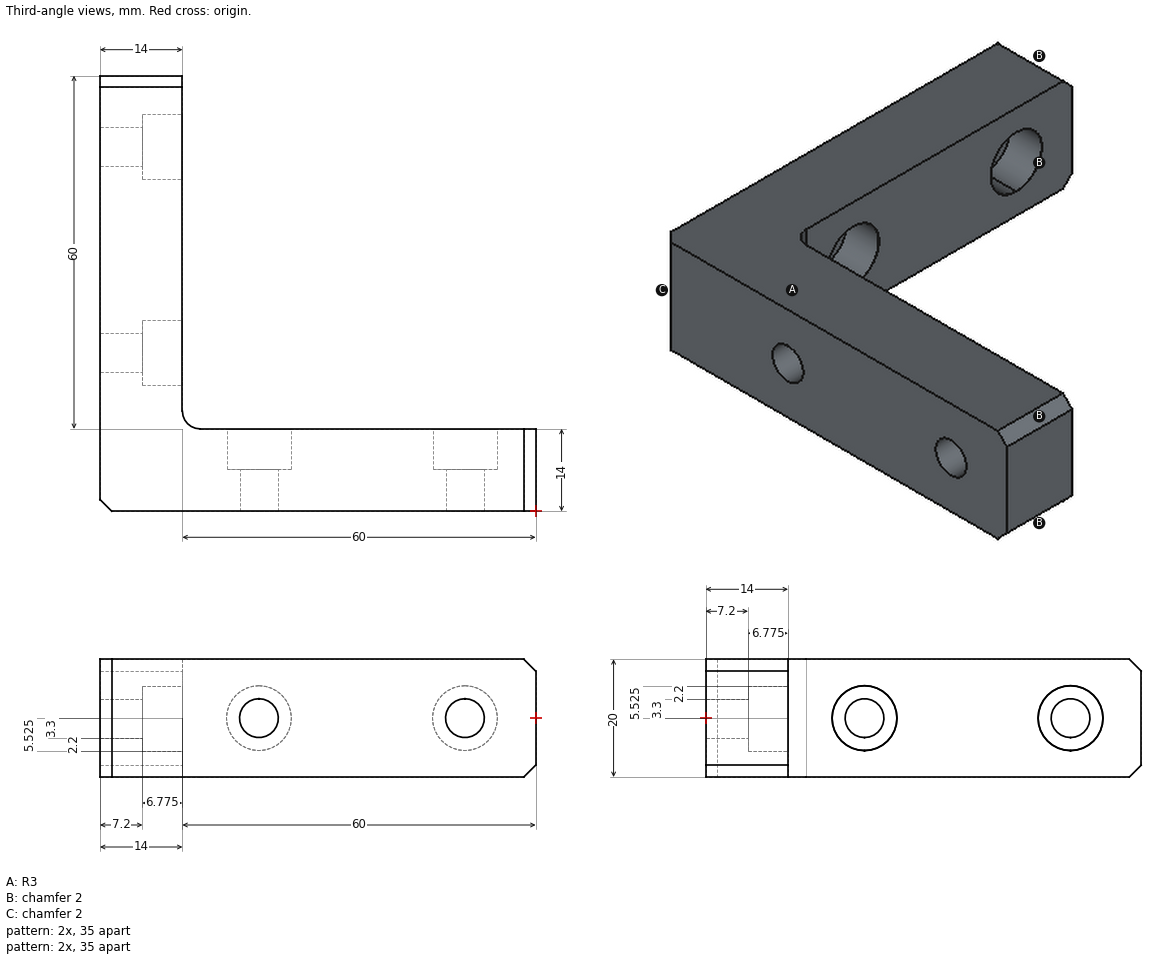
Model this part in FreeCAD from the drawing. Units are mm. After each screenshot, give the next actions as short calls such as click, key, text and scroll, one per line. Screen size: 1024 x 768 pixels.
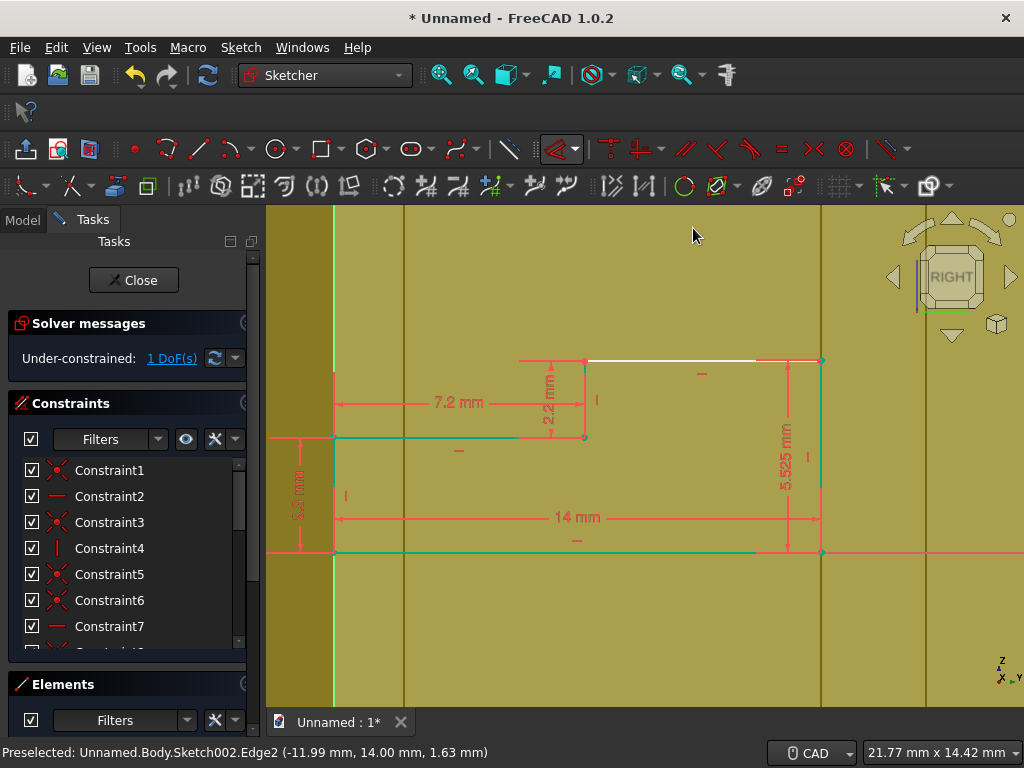
click(750, 361)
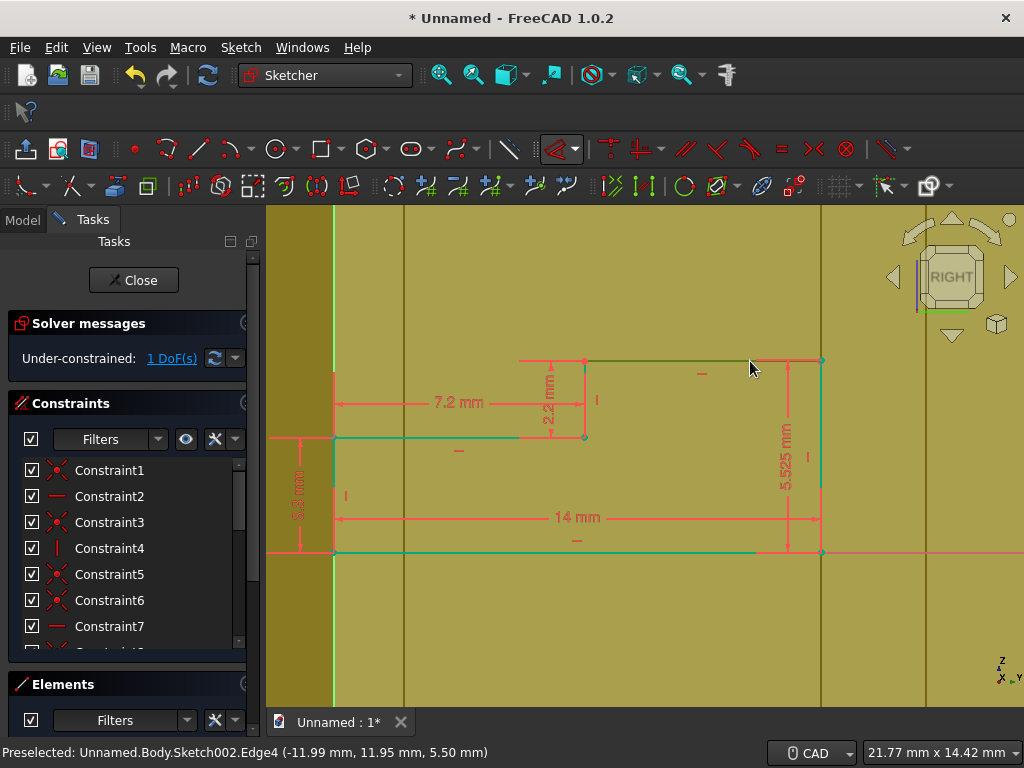
click(578, 150)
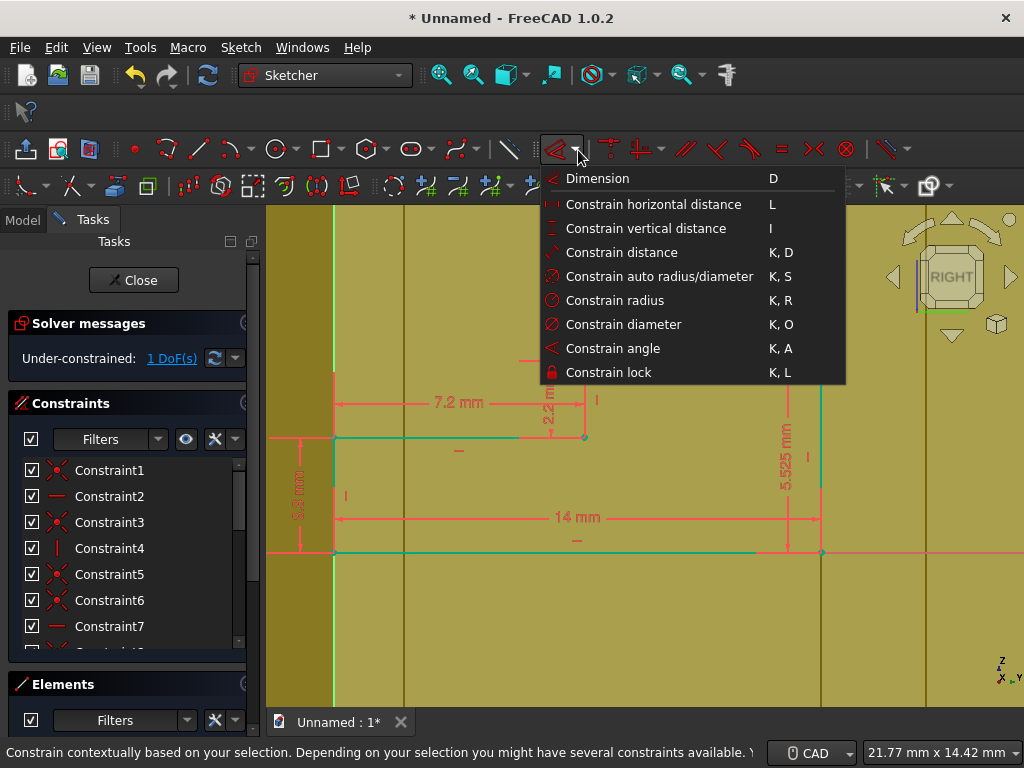
click(693, 204)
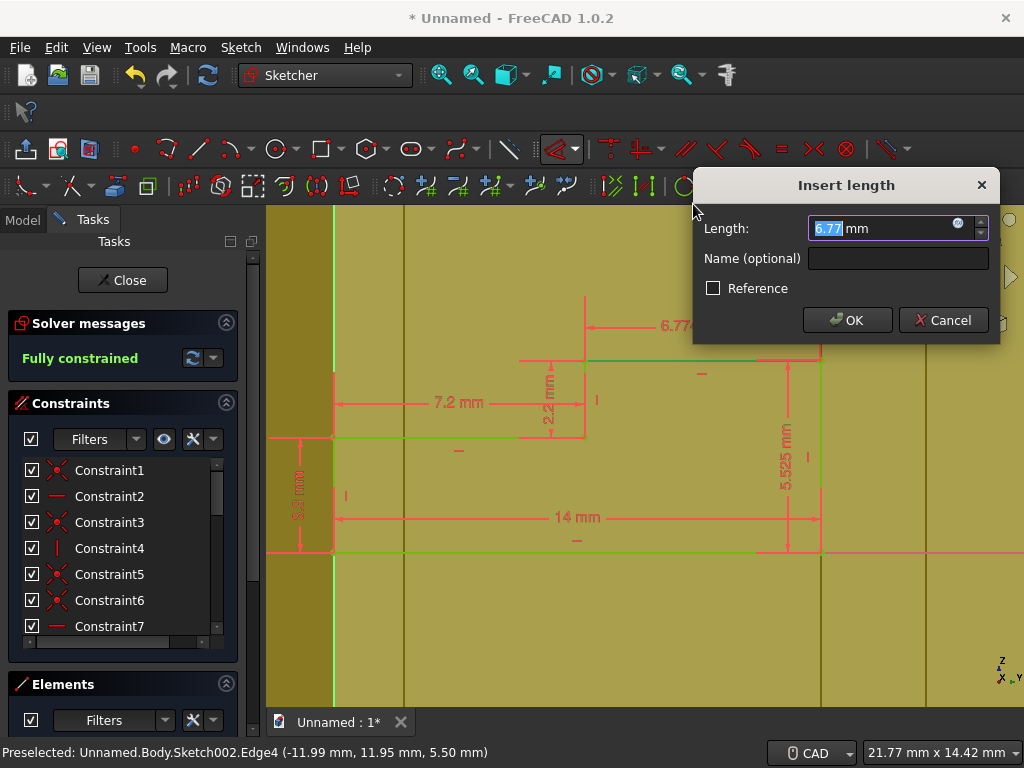
text(6.775)
key(Return)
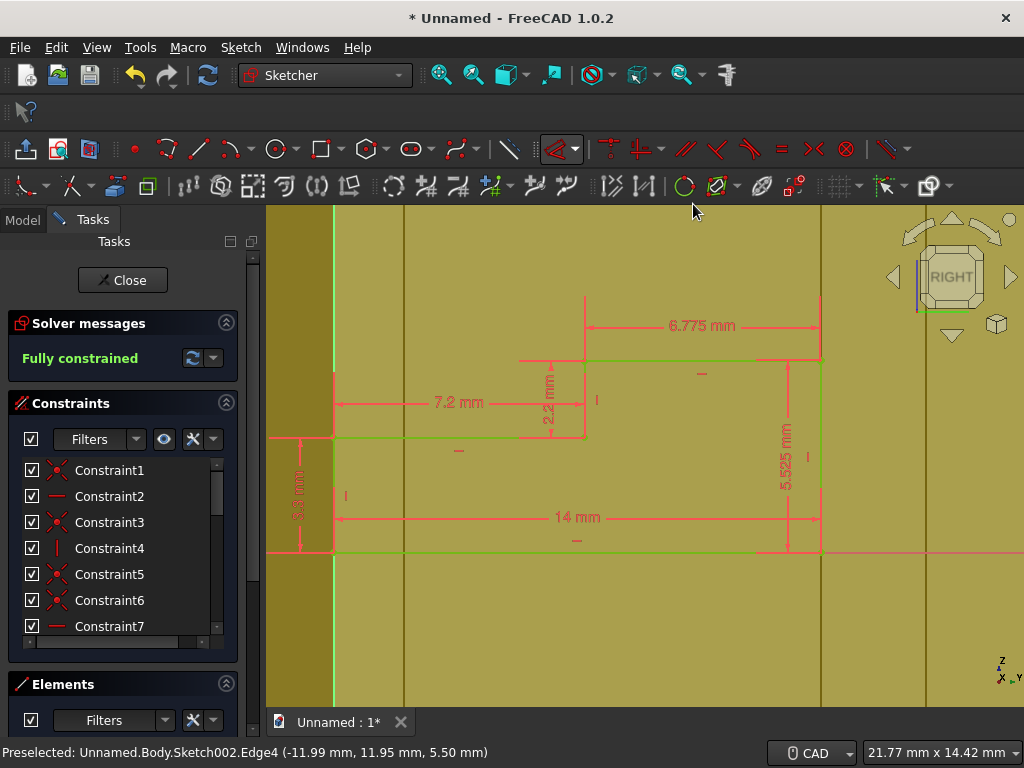
click(123, 280)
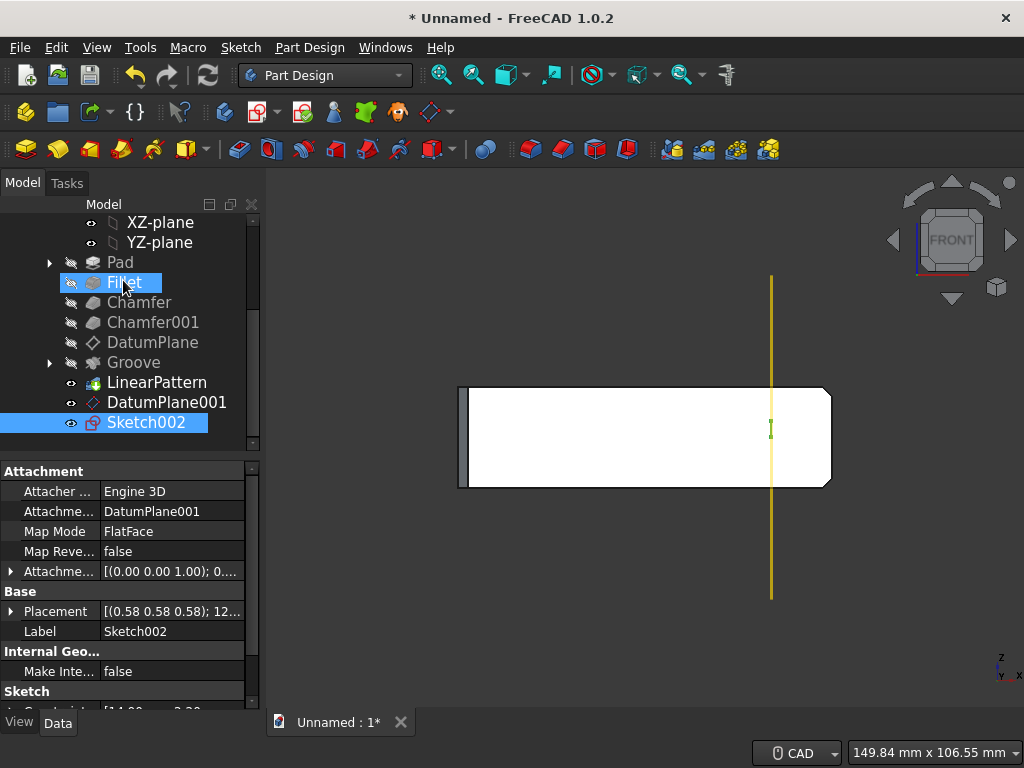
click(304, 150)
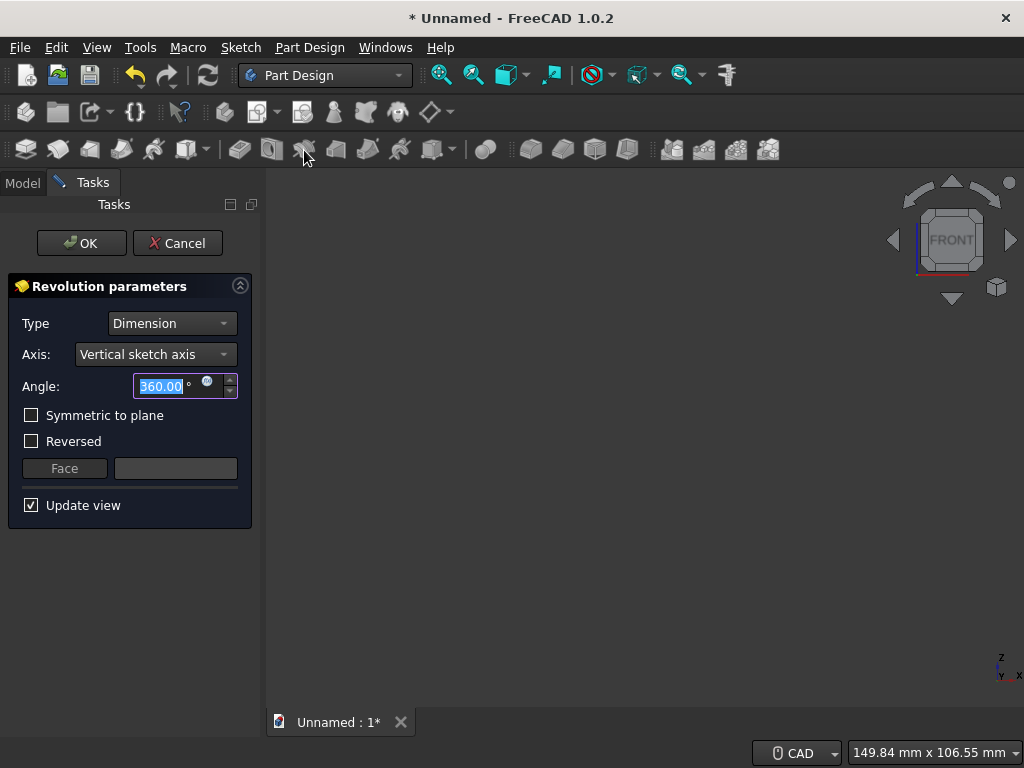
click(156, 354)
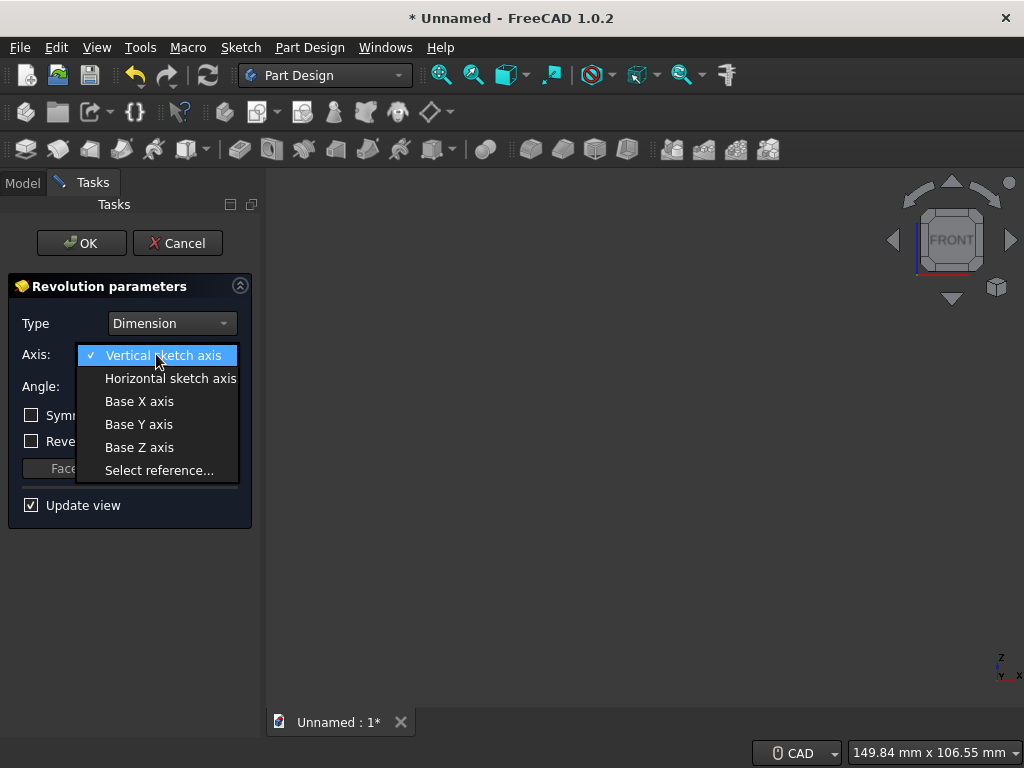
click(156, 378)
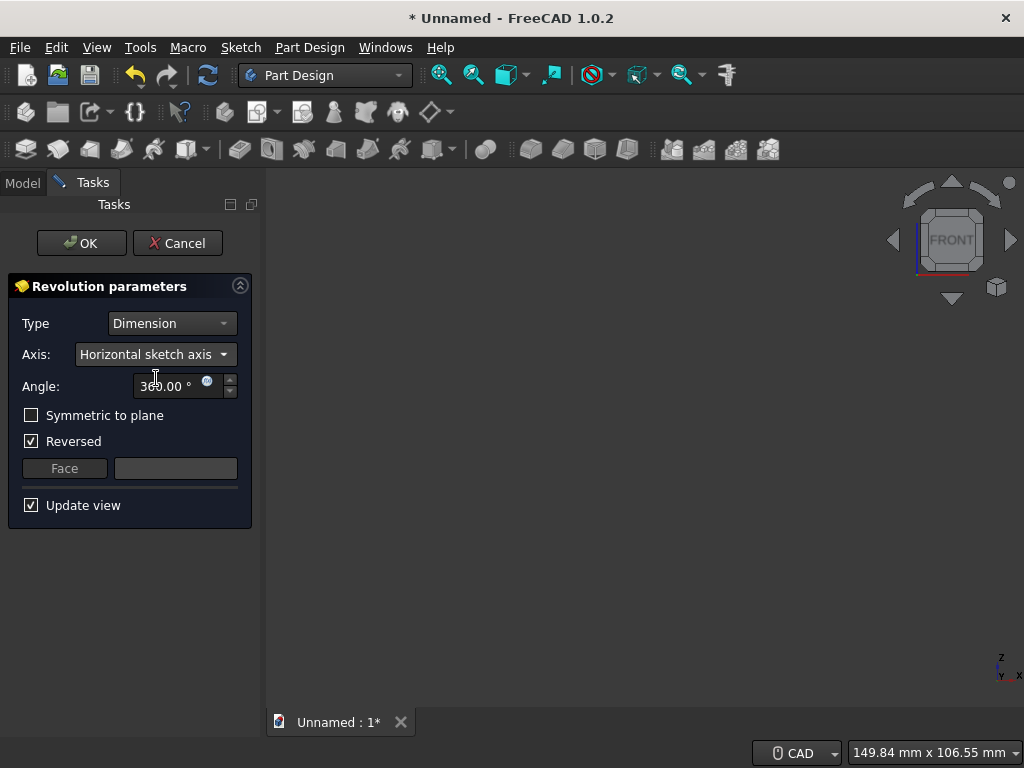
click(82, 243)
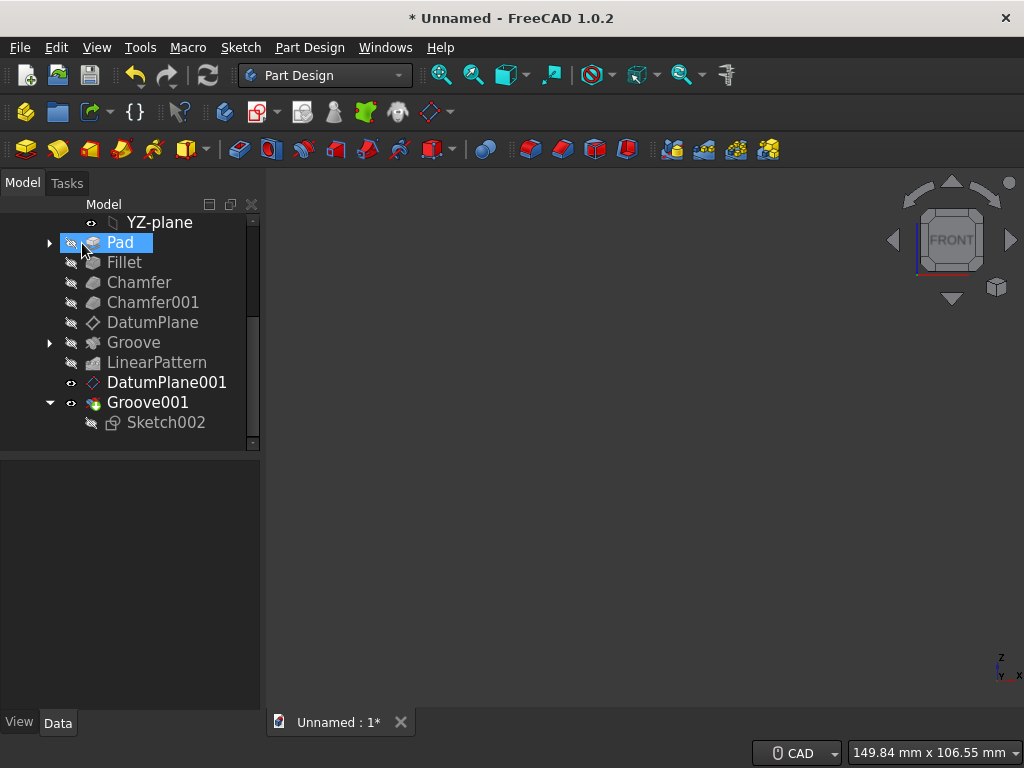
click(116, 383)
key(space)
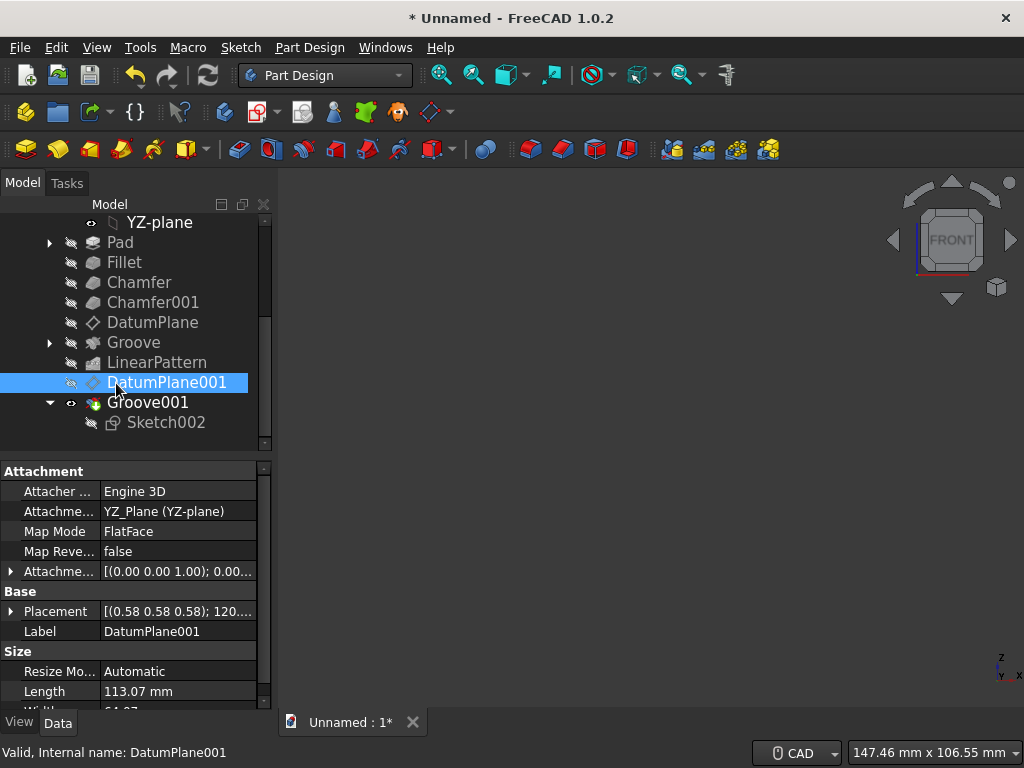
click(442, 76)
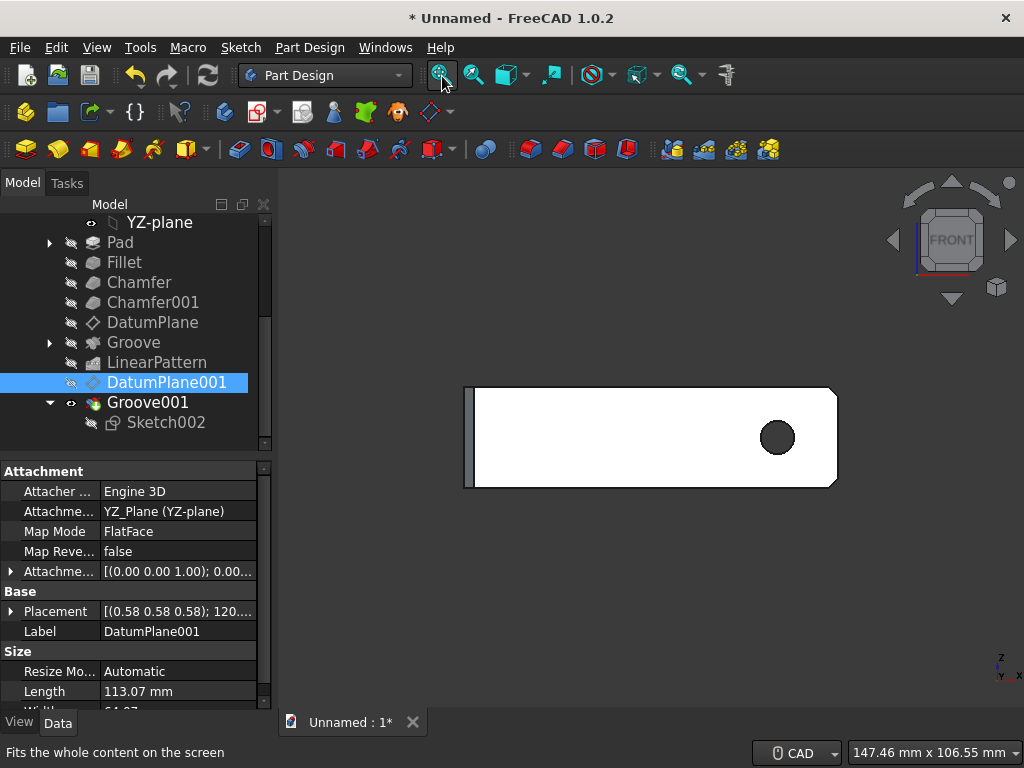
click(116, 403)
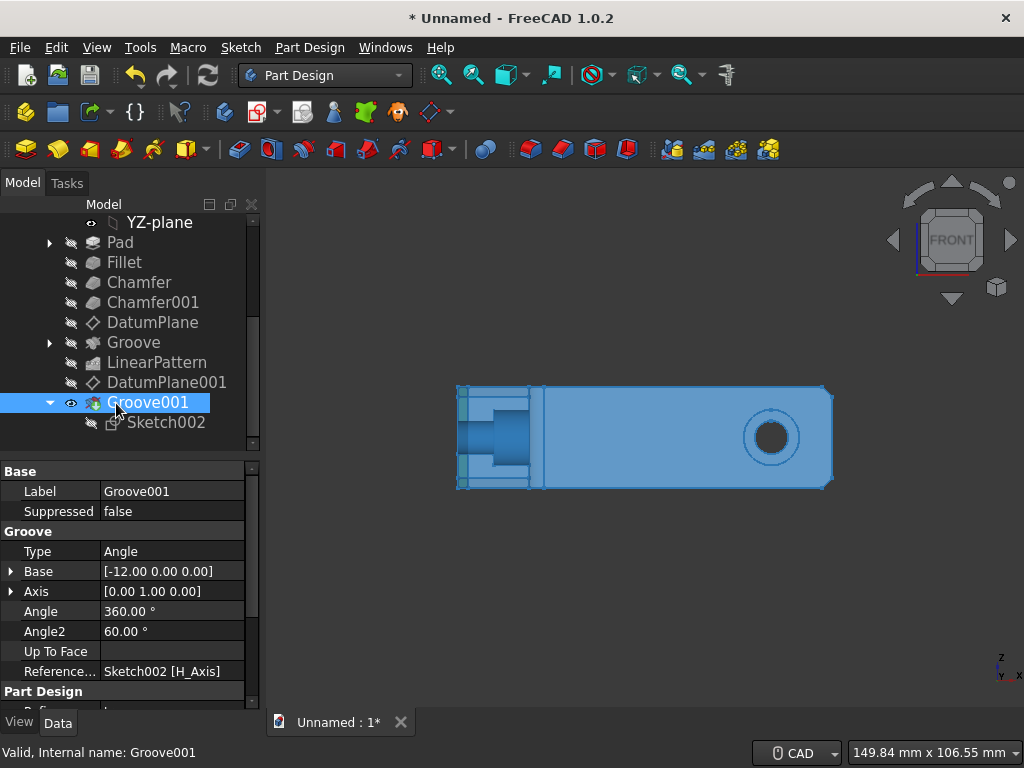
click(704, 150)